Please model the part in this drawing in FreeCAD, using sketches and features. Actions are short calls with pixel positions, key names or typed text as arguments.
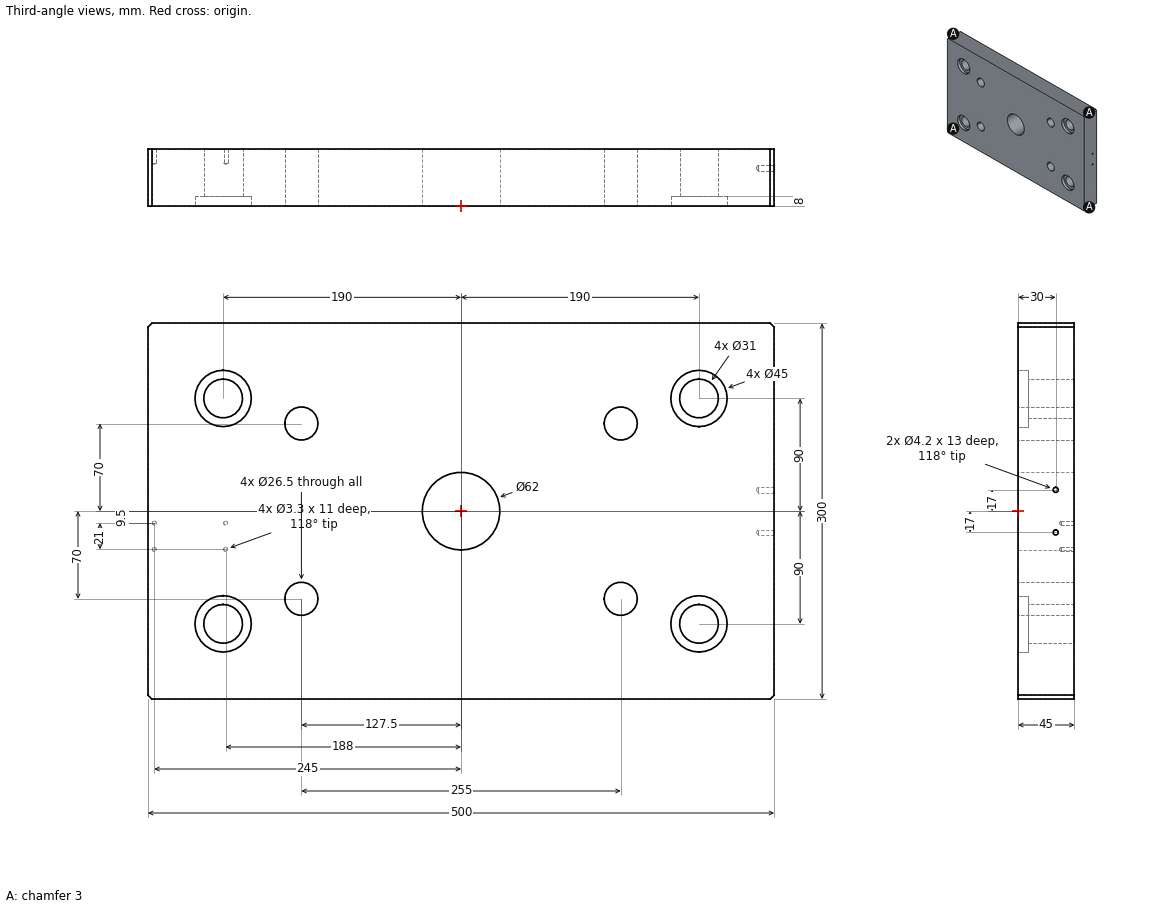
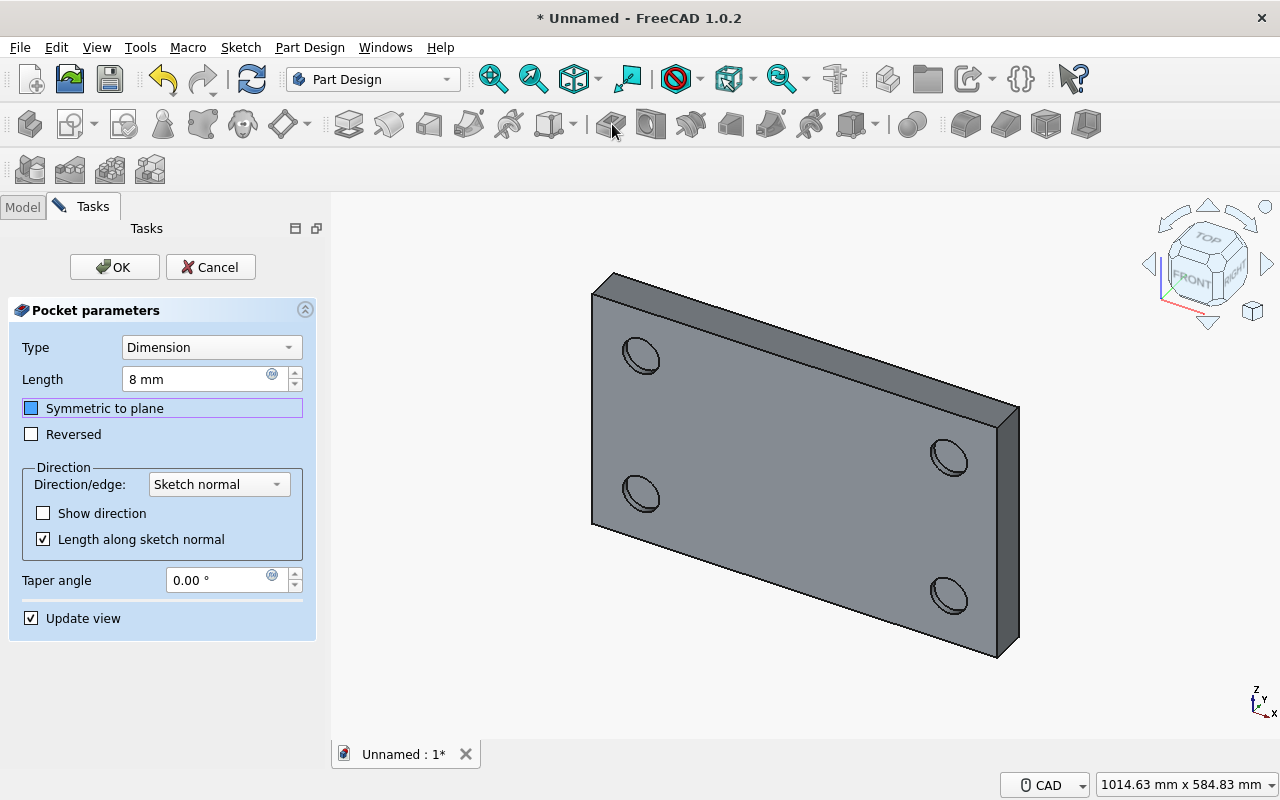
click(115, 267)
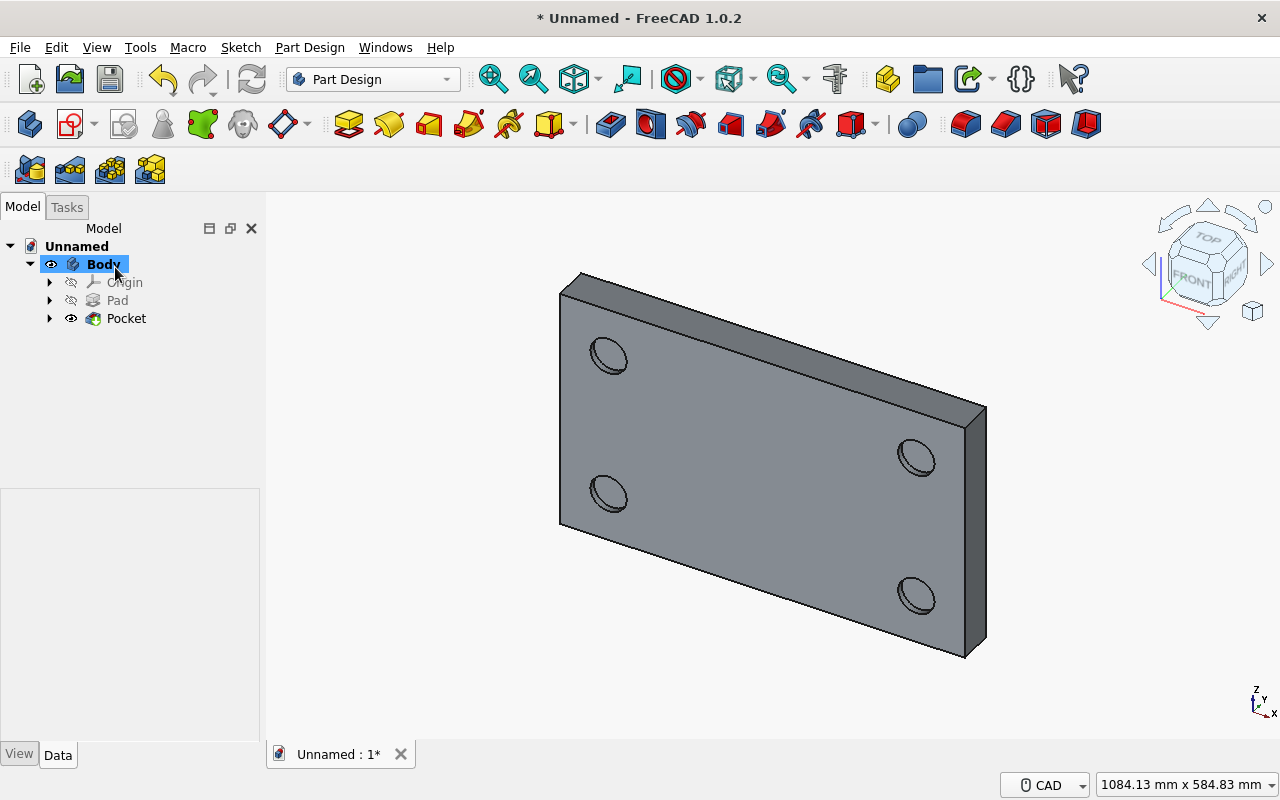
click(976, 417)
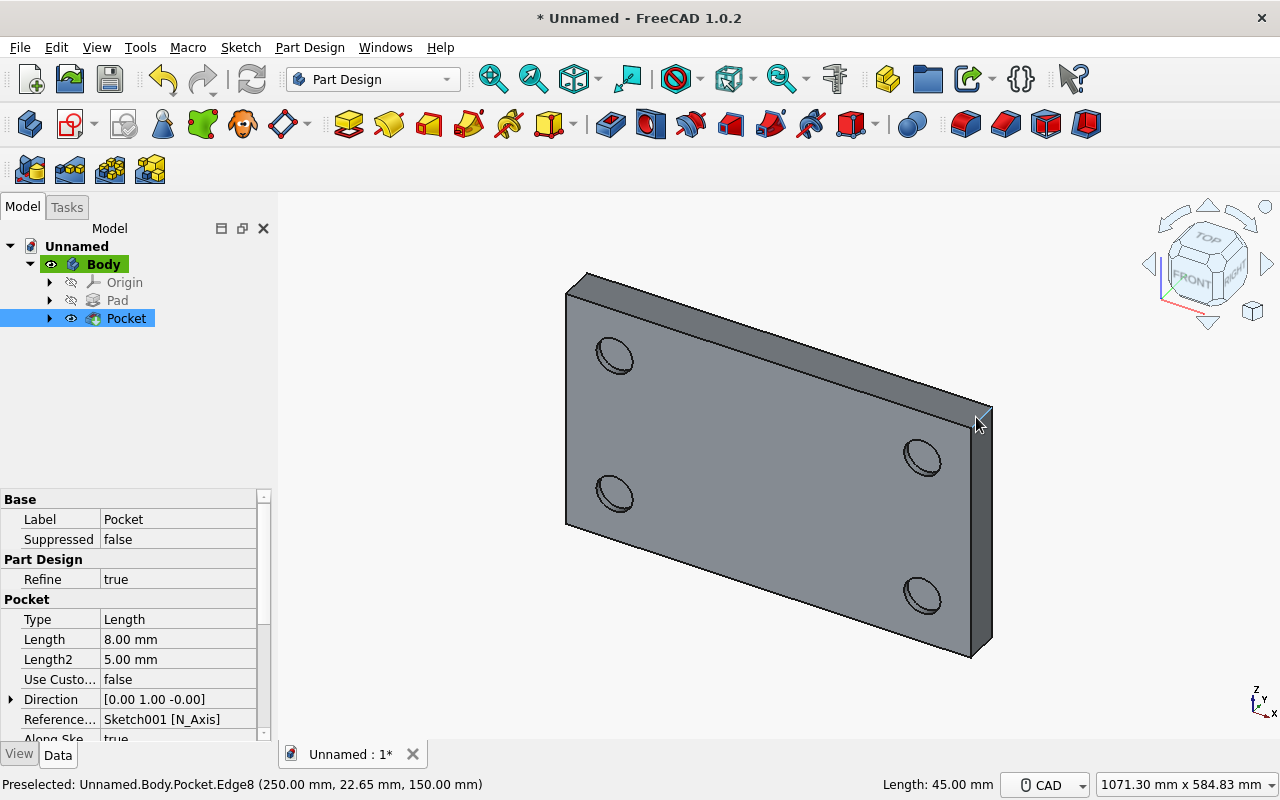
key(0)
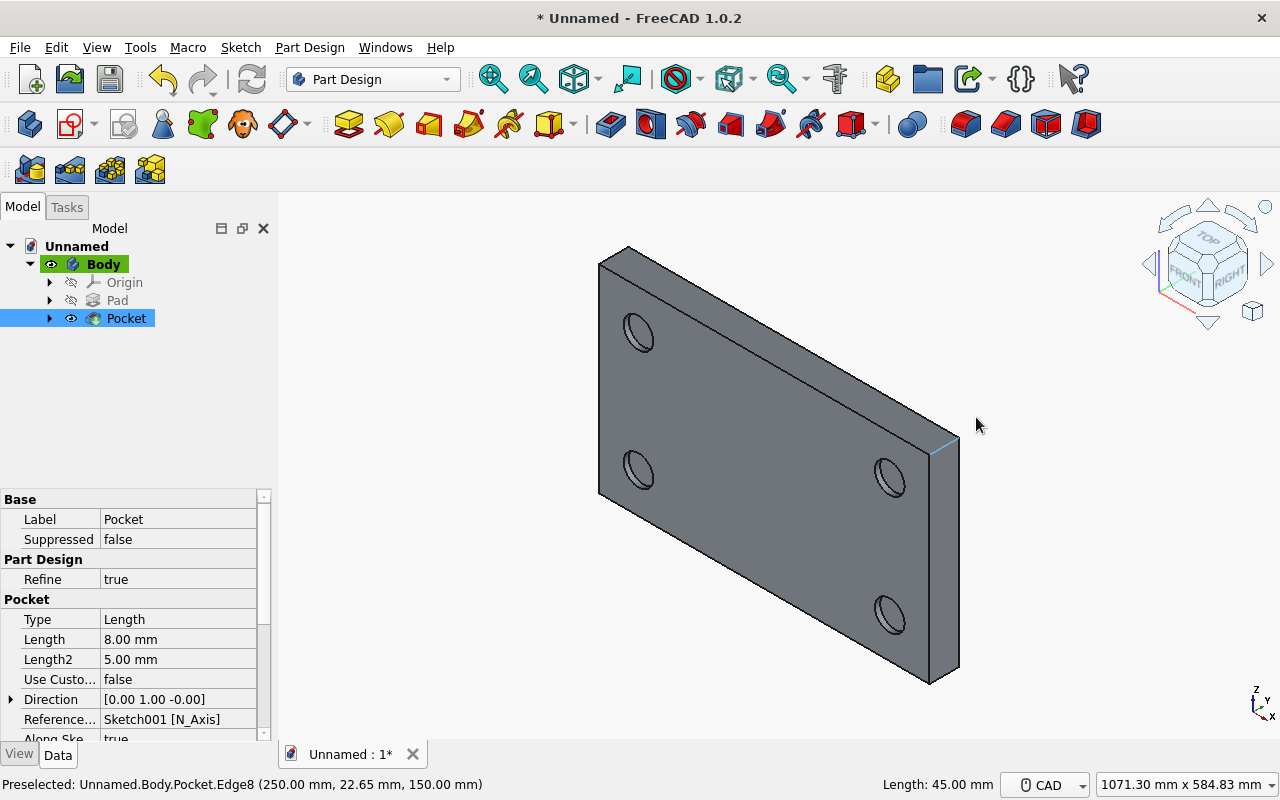
key(2)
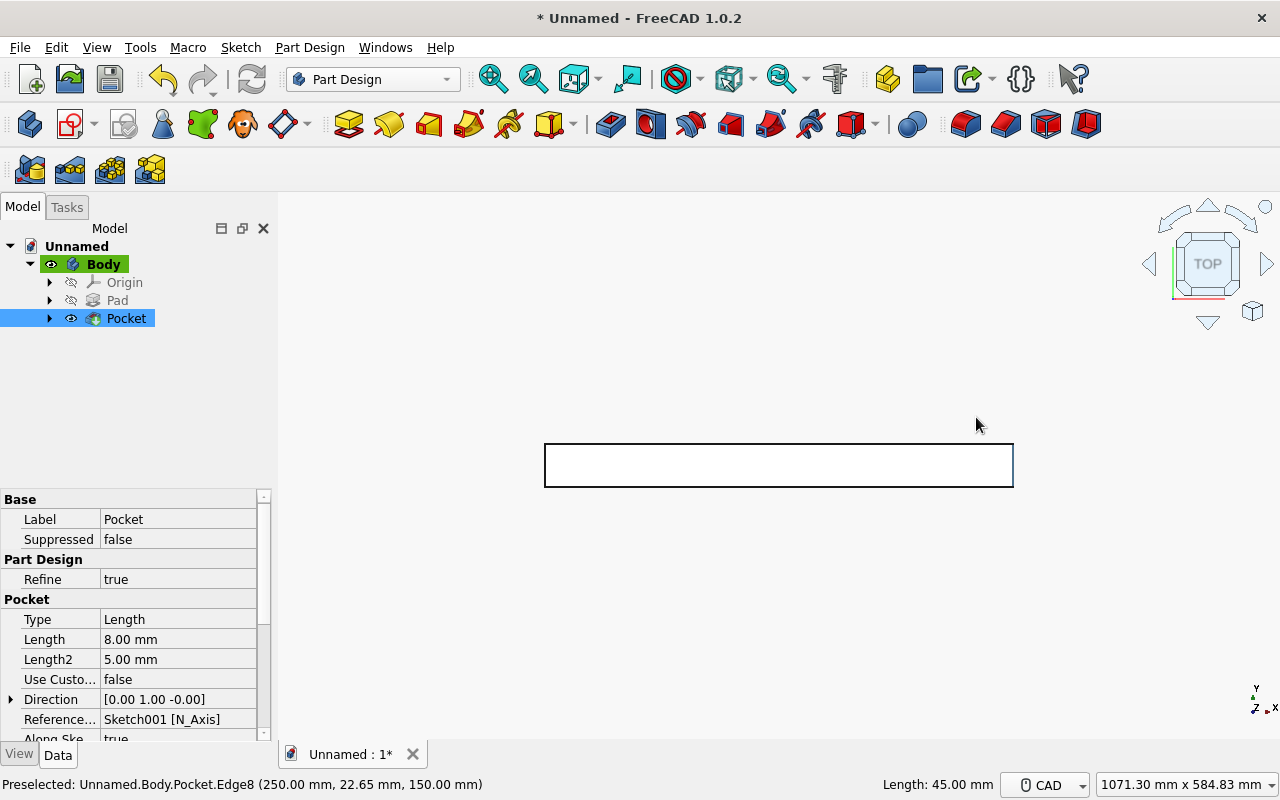
click(545, 465, ctrl)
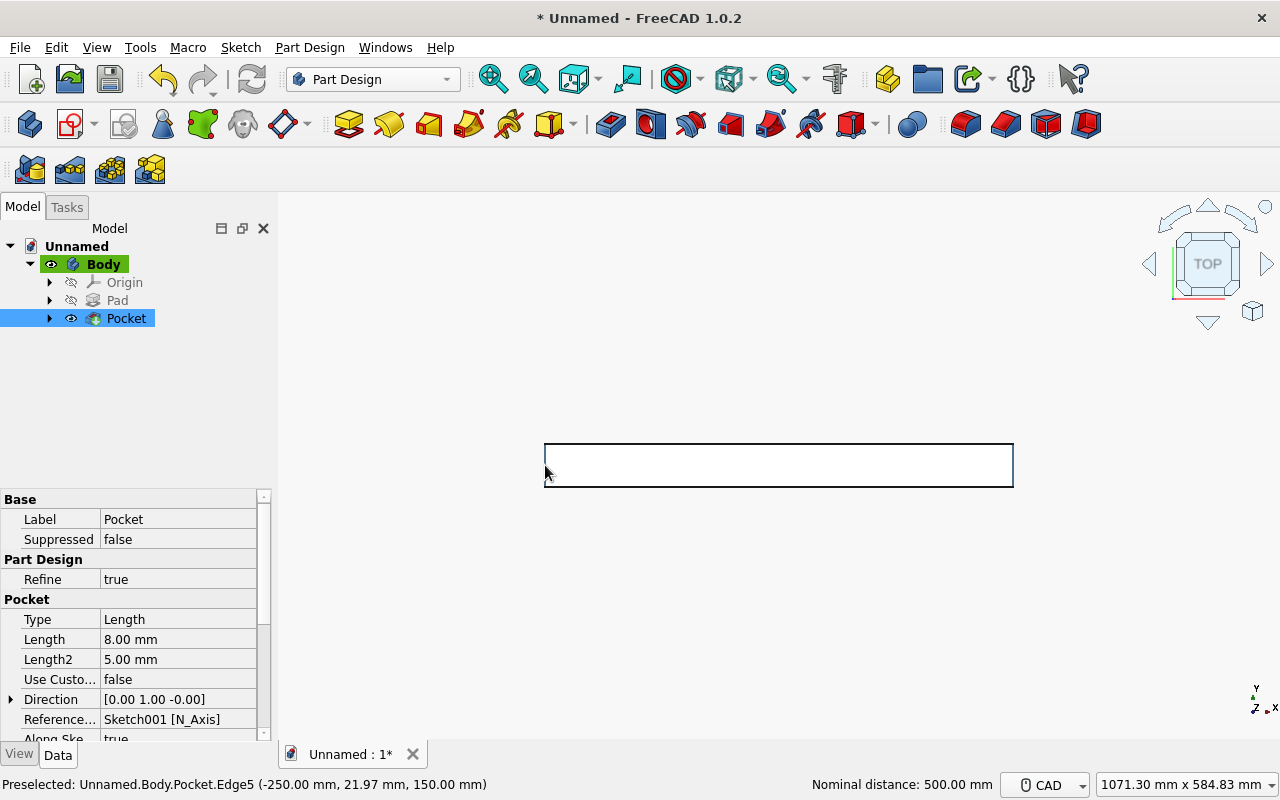
key(1)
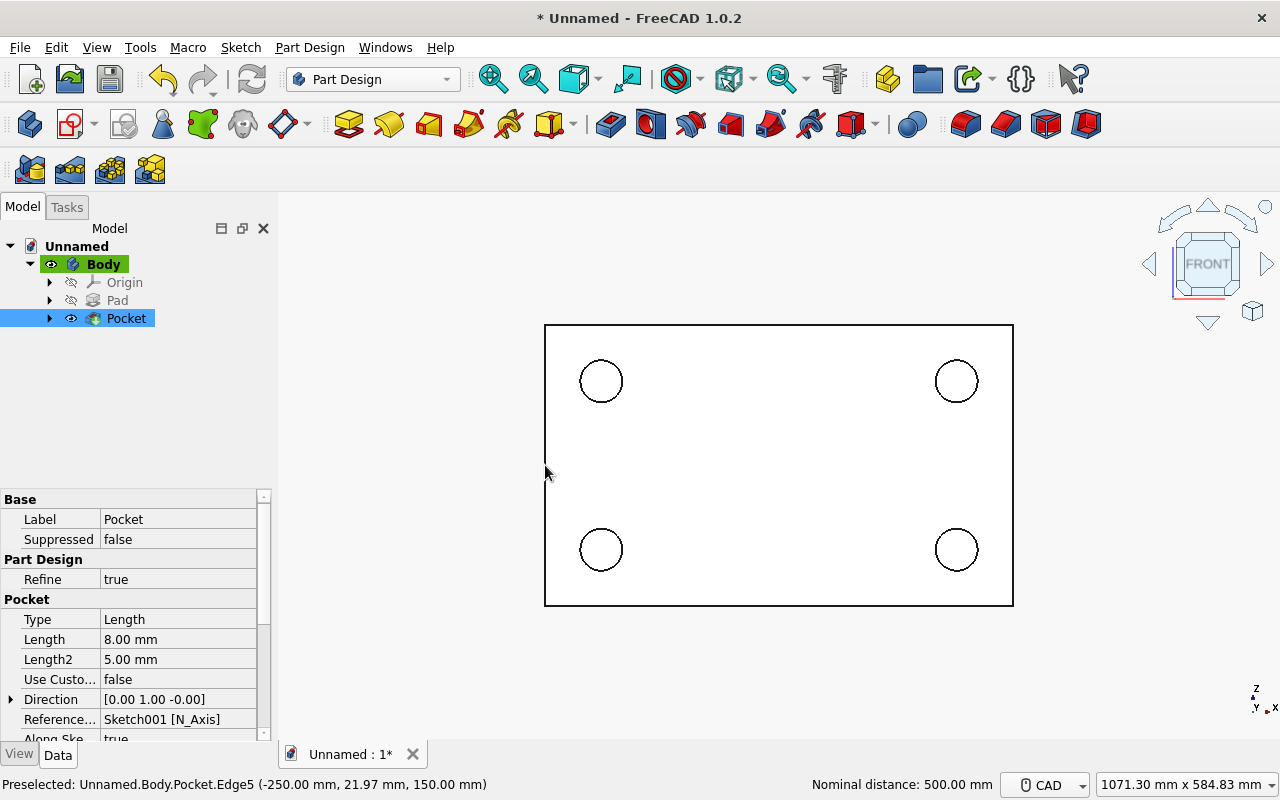
key(3)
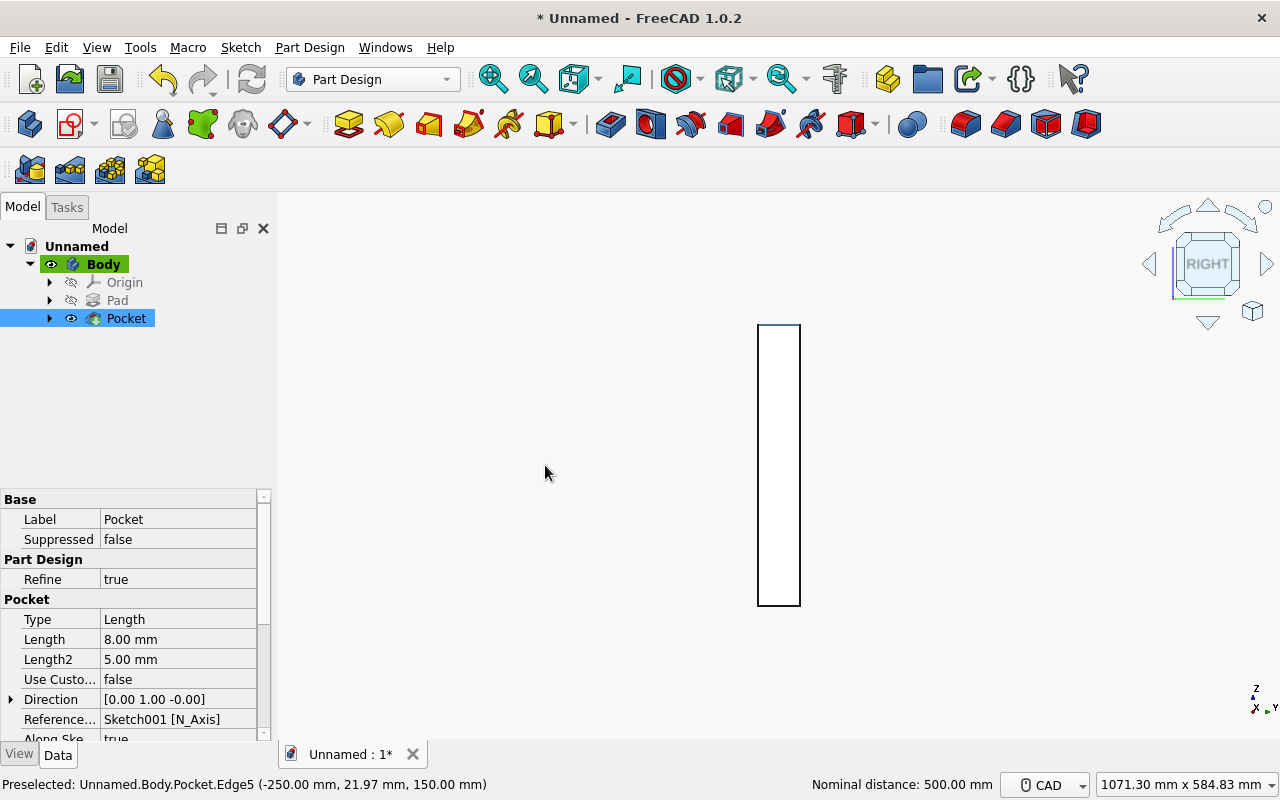
click(779, 605, ctrl)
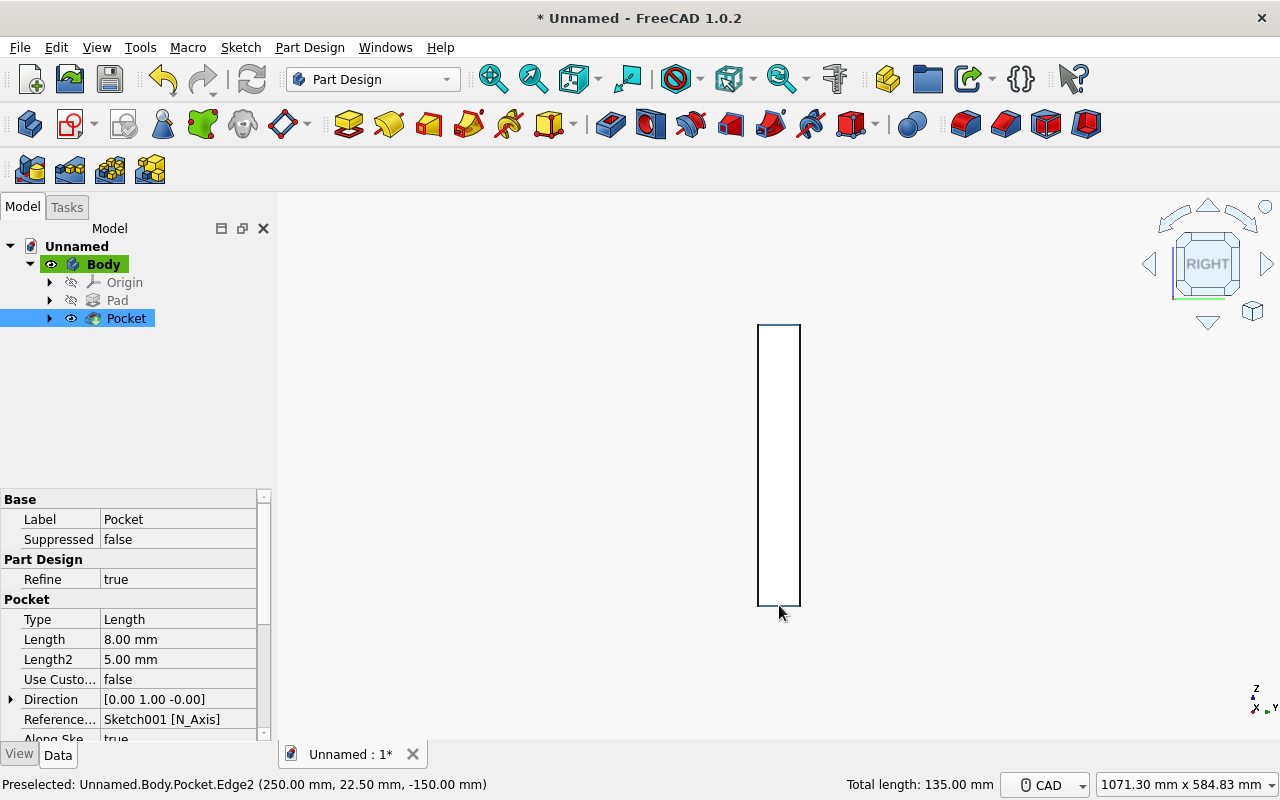
key(5)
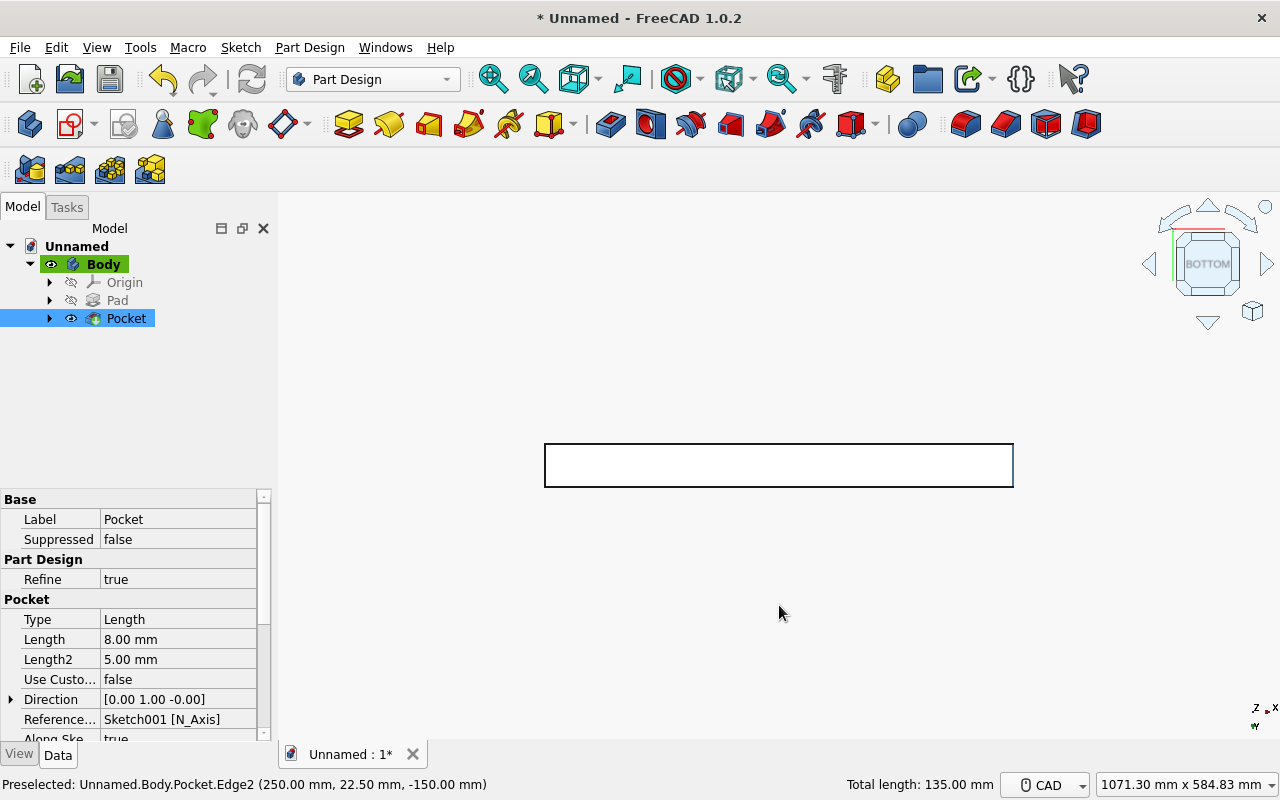
click(545, 464, ctrl)